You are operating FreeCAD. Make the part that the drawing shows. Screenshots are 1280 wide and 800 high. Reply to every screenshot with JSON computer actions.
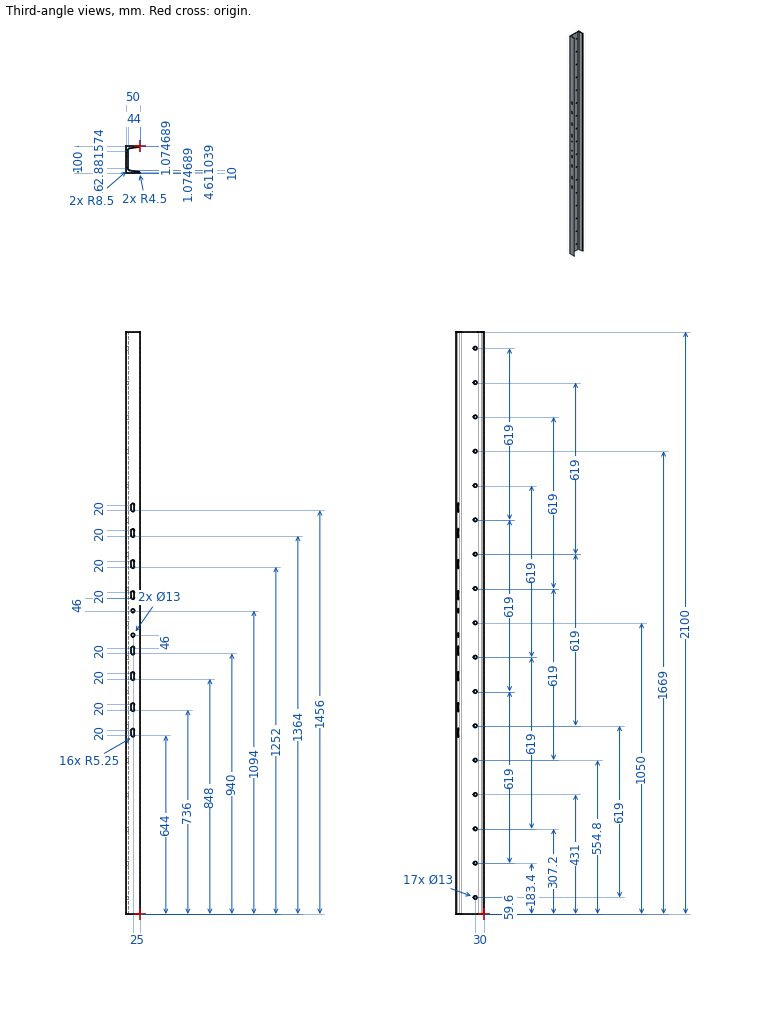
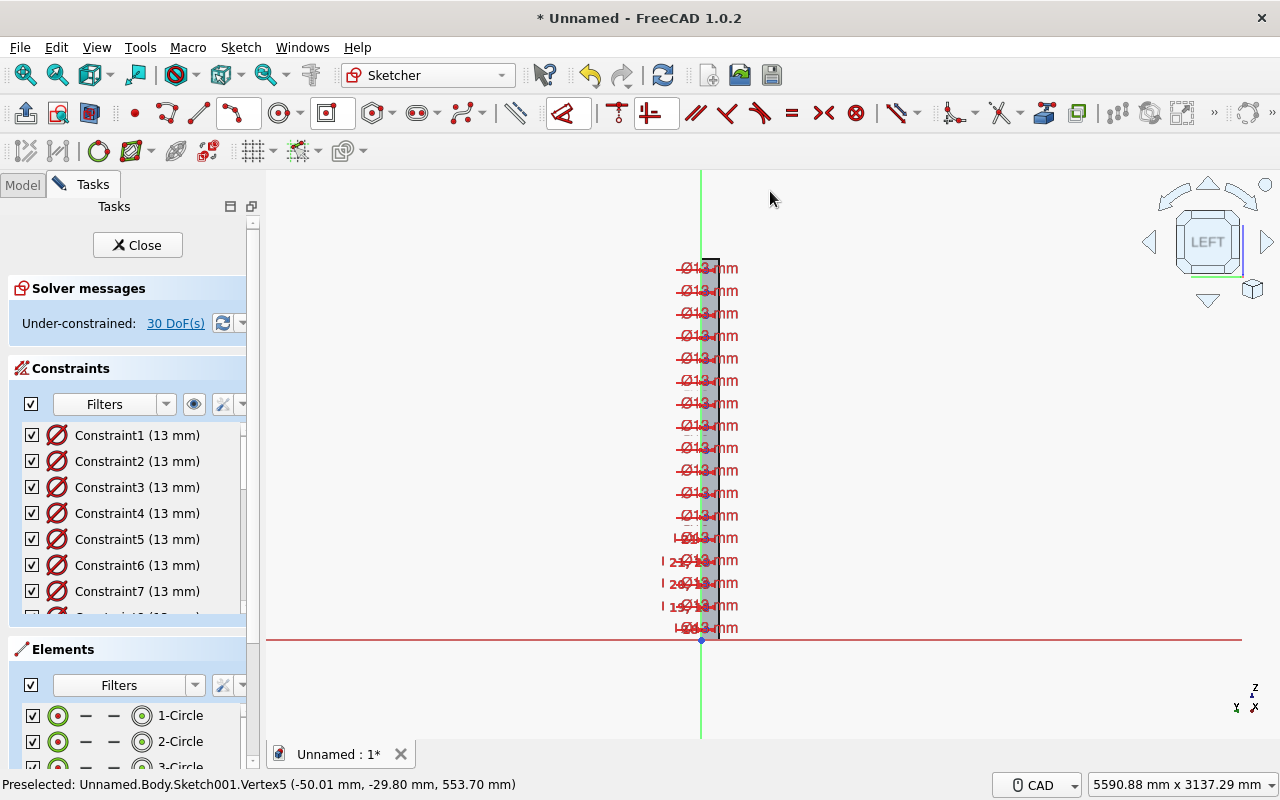
{"action": "left_click", "coordinate": [707, 540]}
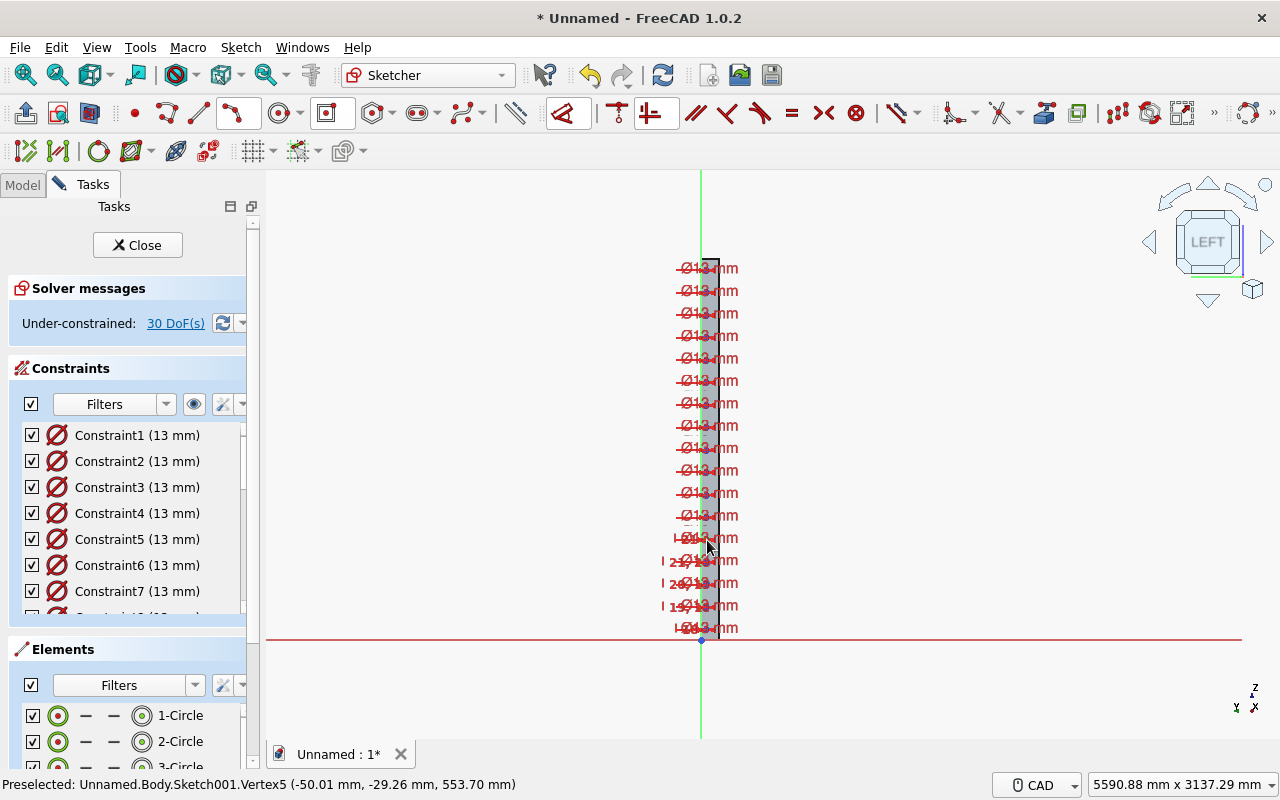
{"action": "left_click", "coordinate": [707, 518]}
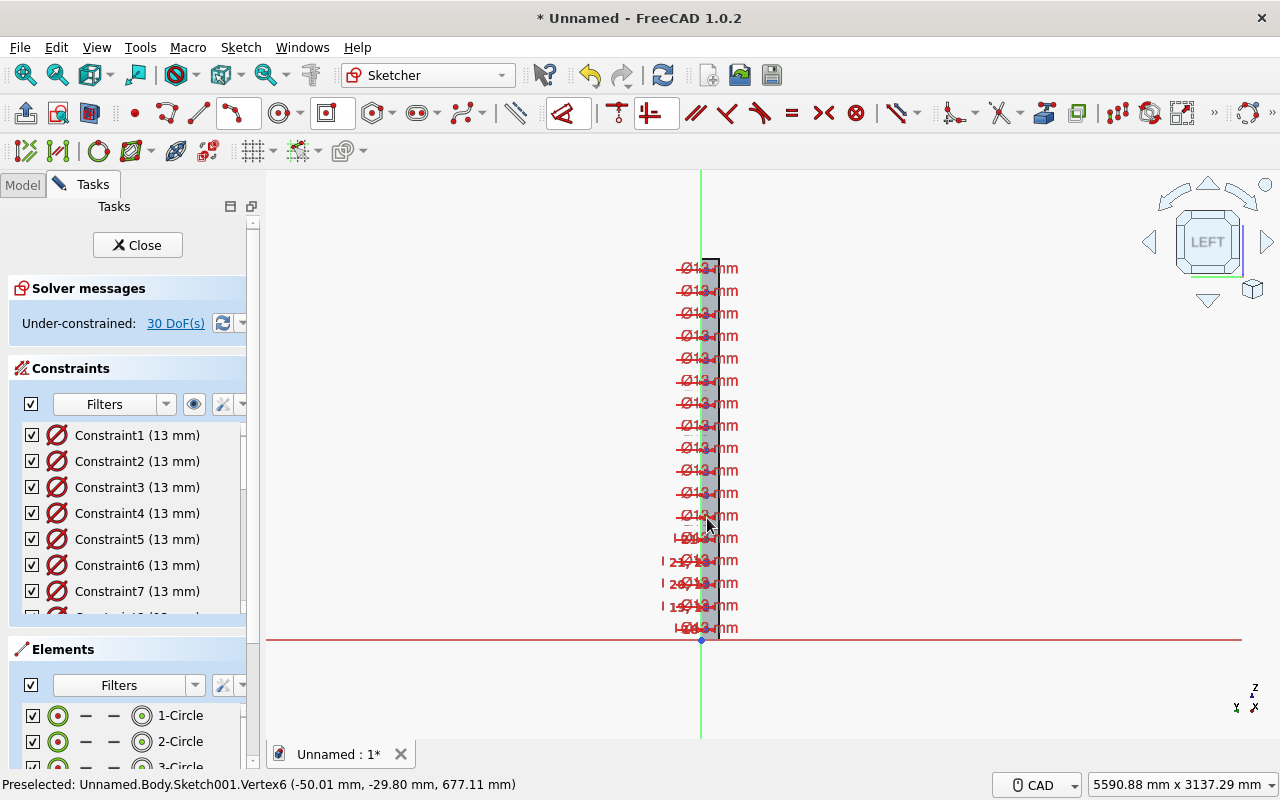
{"action": "key", "text": "v"}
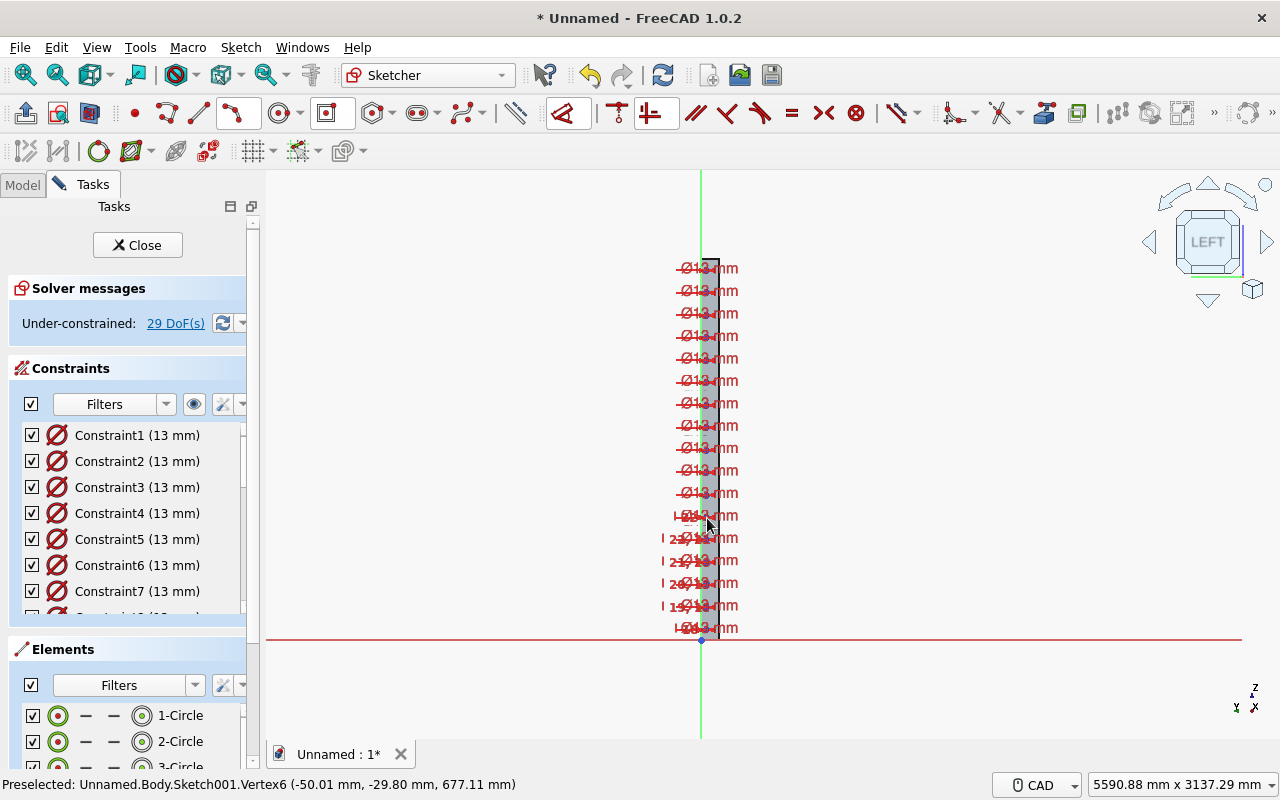
{"action": "left_click", "coordinate": [707, 518]}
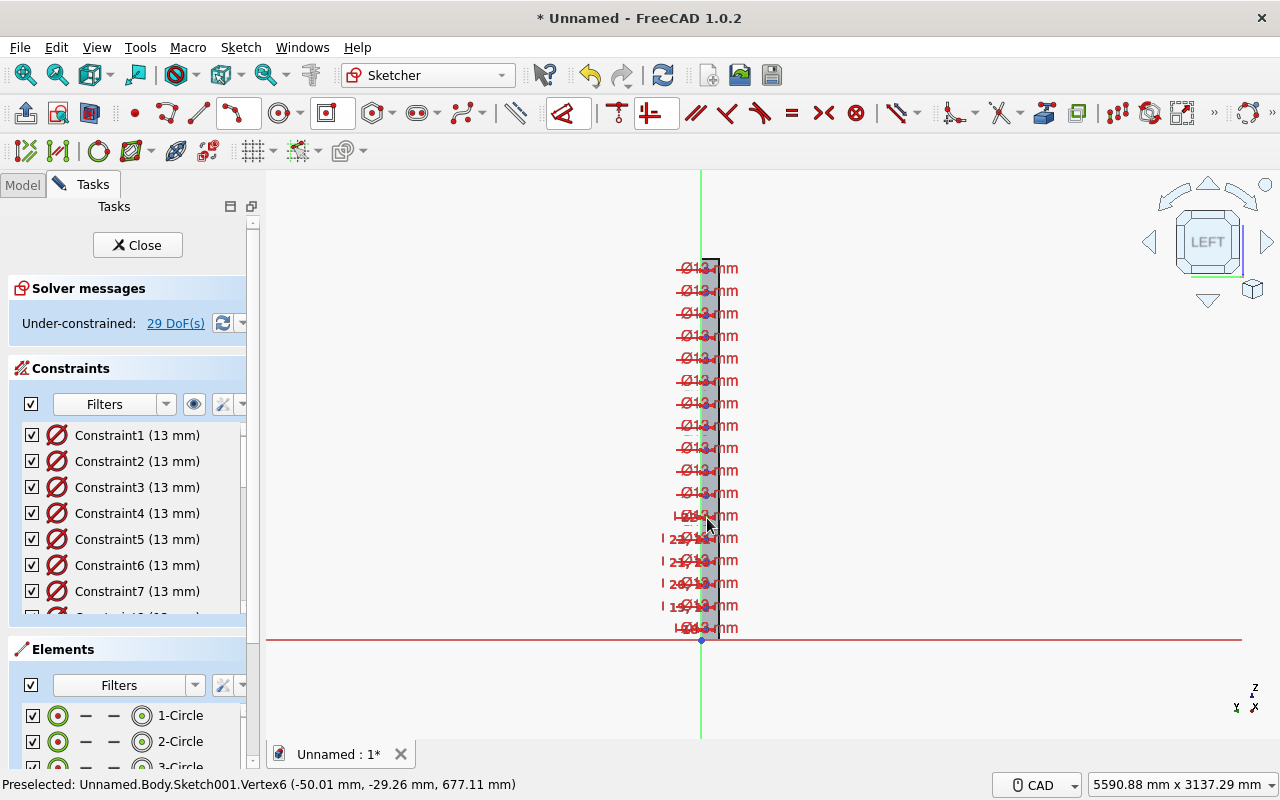
{"action": "left_click", "coordinate": [707, 495]}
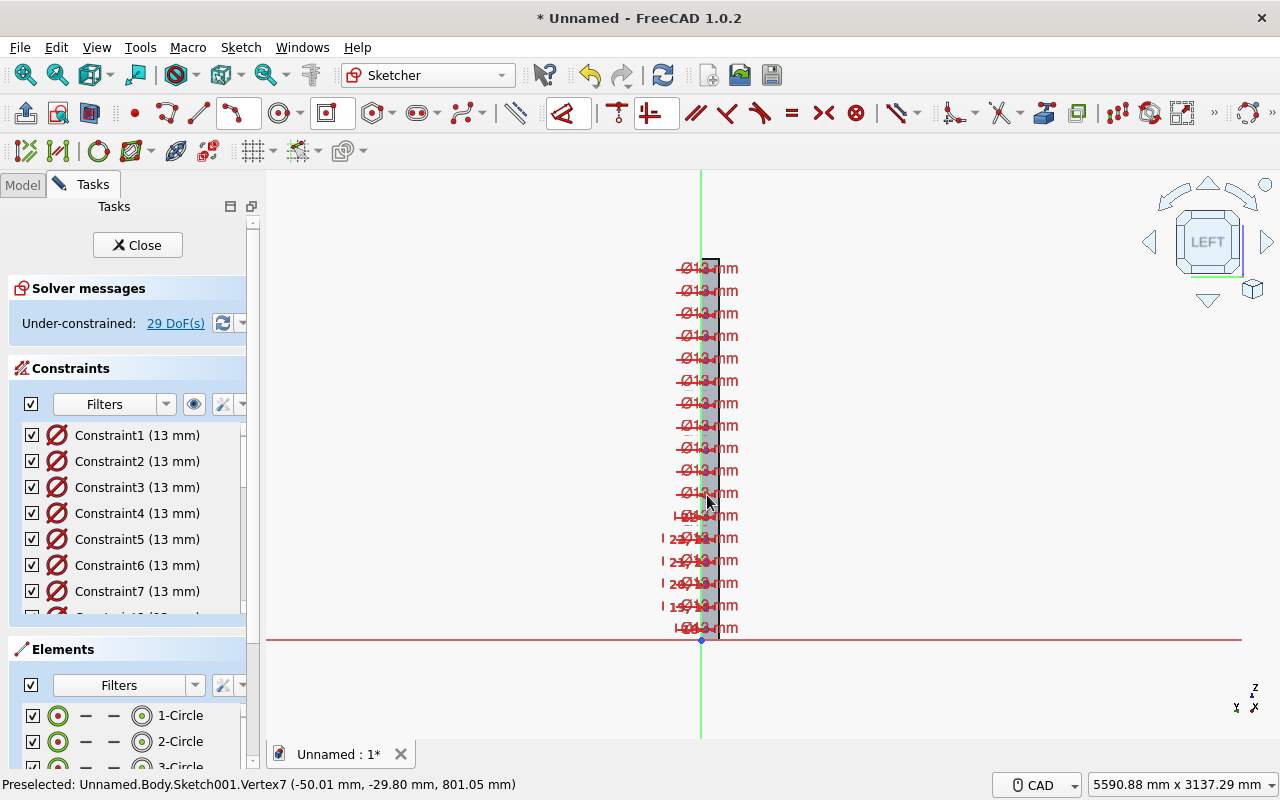
{"action": "key", "text": "v"}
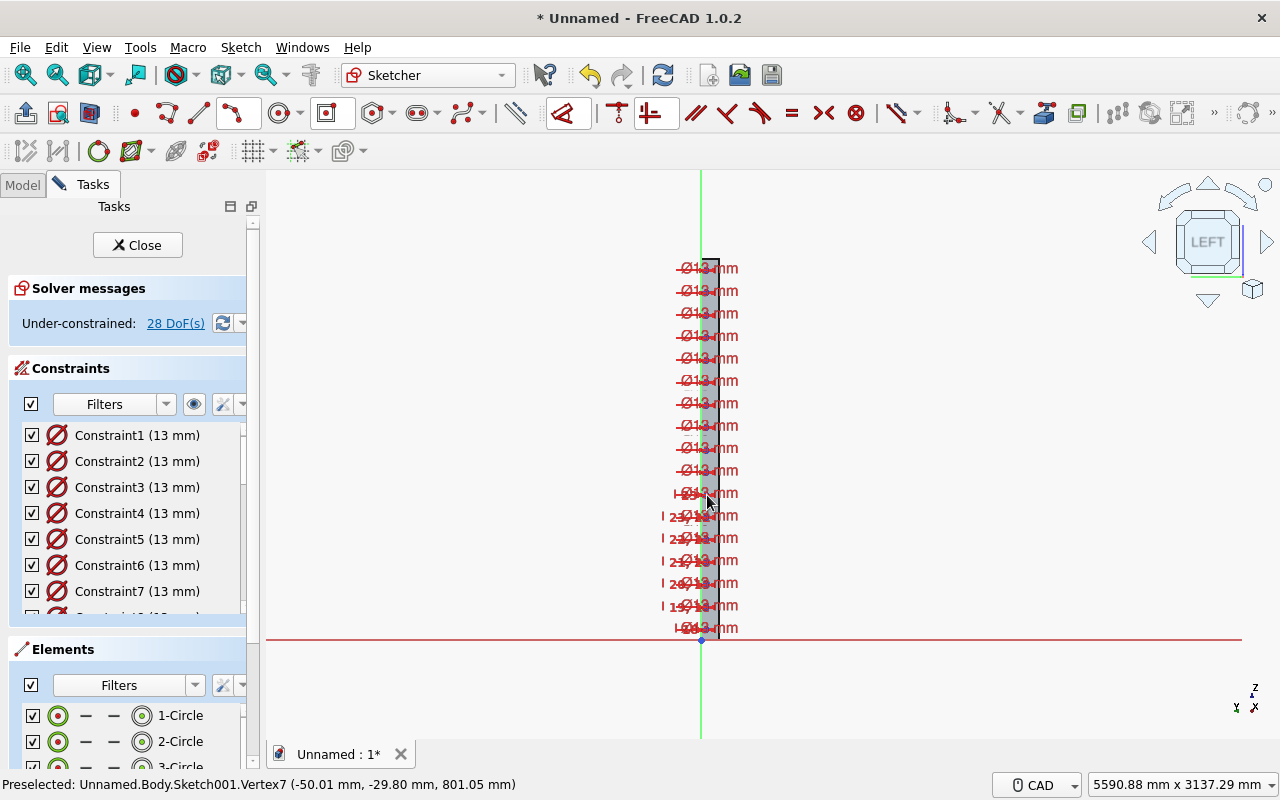
{"action": "left_click", "coordinate": [707, 495]}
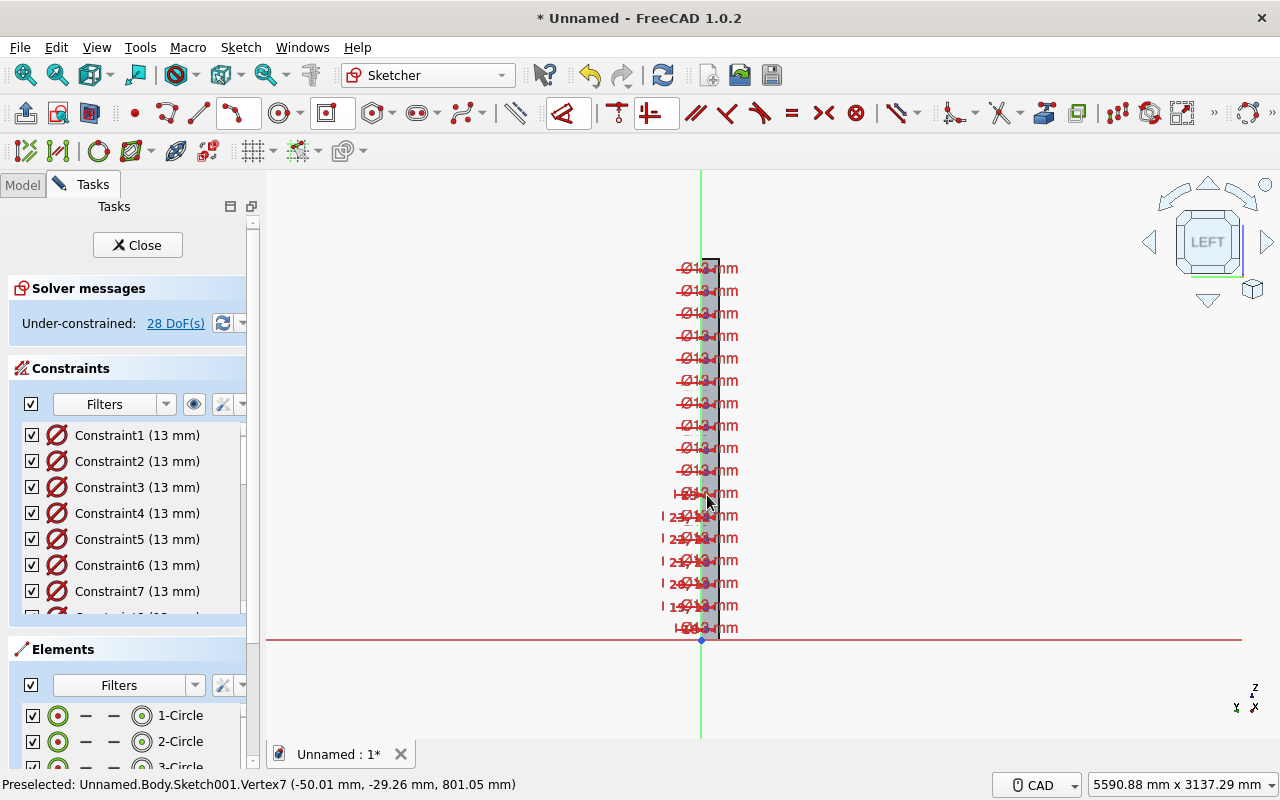
{"action": "left_click", "coordinate": [707, 472]}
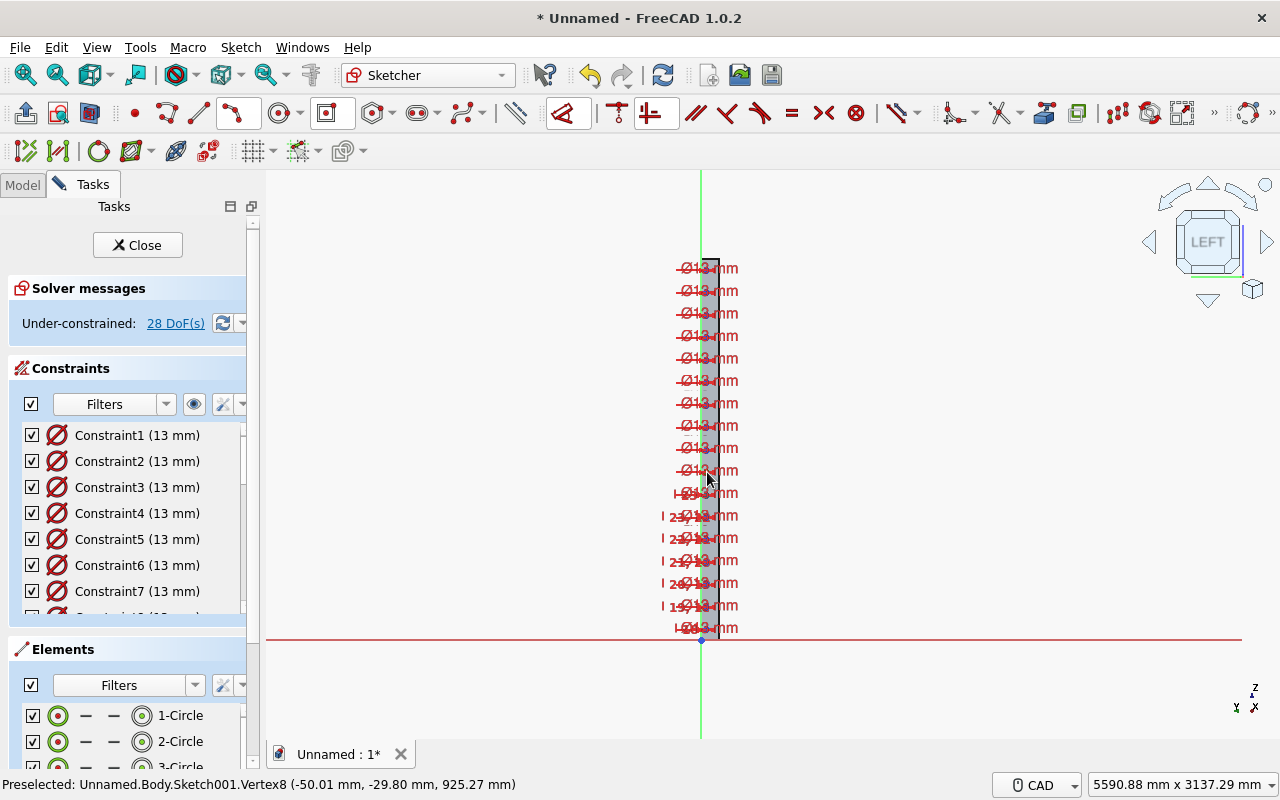
{"action": "left_click", "coordinate": [674, 114]}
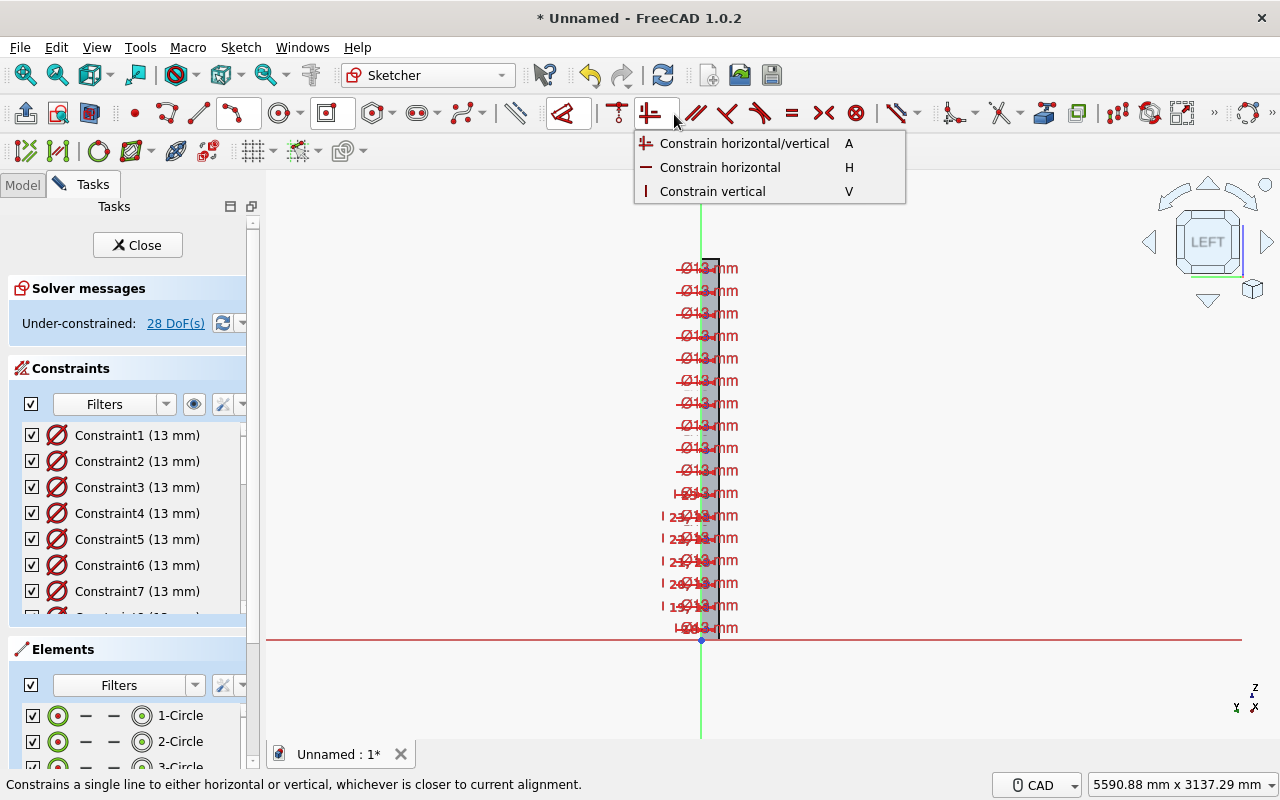
{"action": "left_click", "coordinate": [770, 191]}